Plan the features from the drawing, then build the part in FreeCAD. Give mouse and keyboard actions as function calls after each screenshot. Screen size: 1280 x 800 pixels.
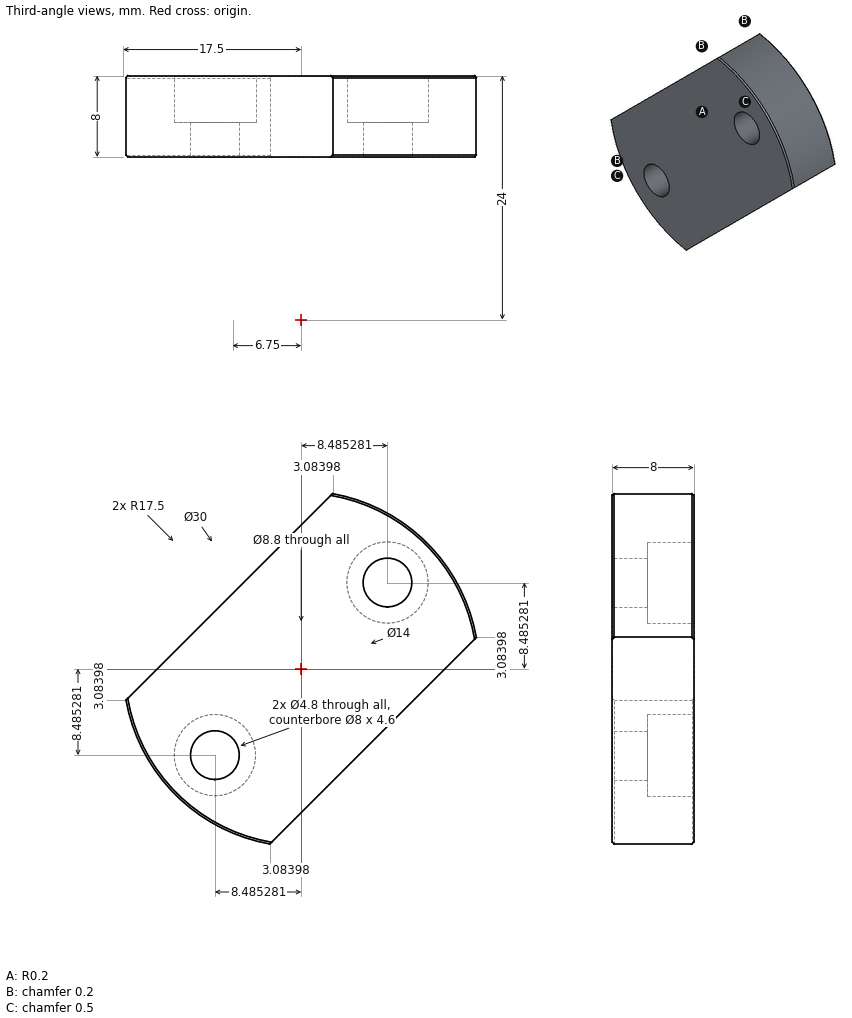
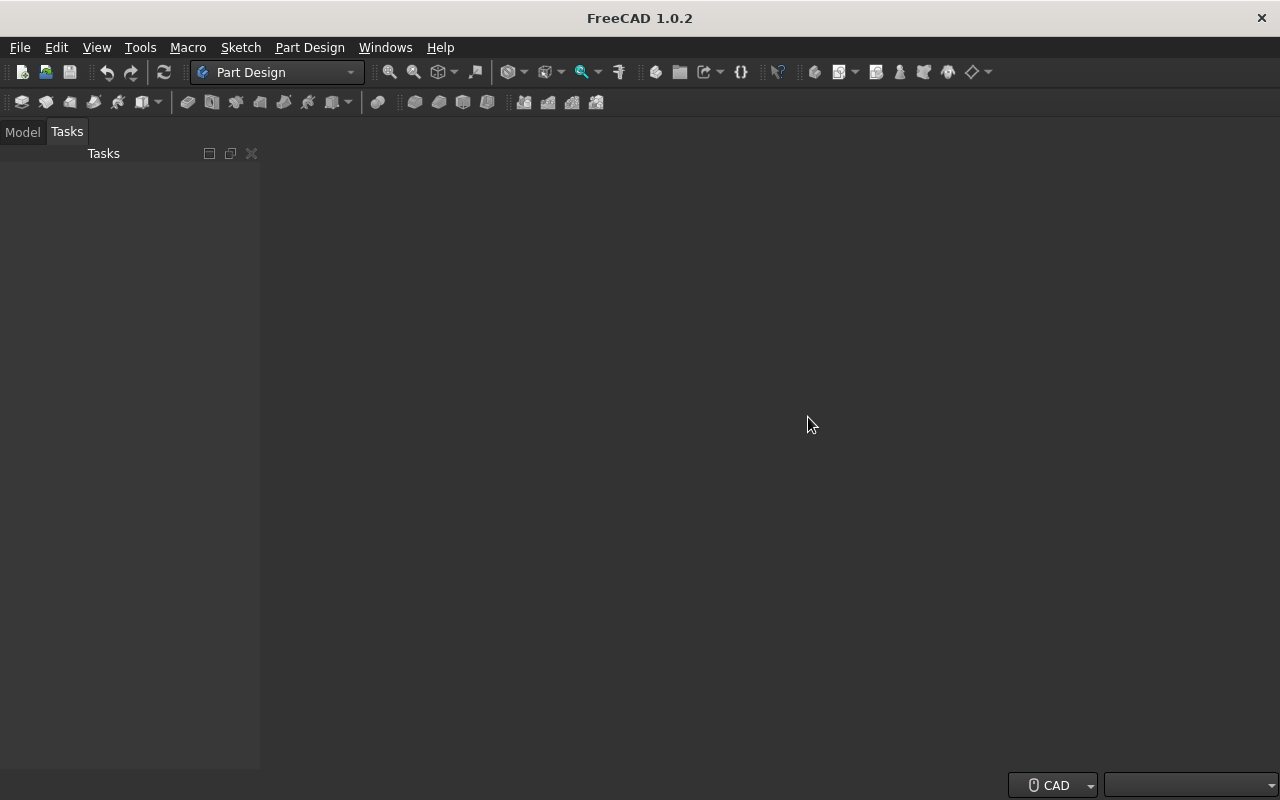
click(22, 72)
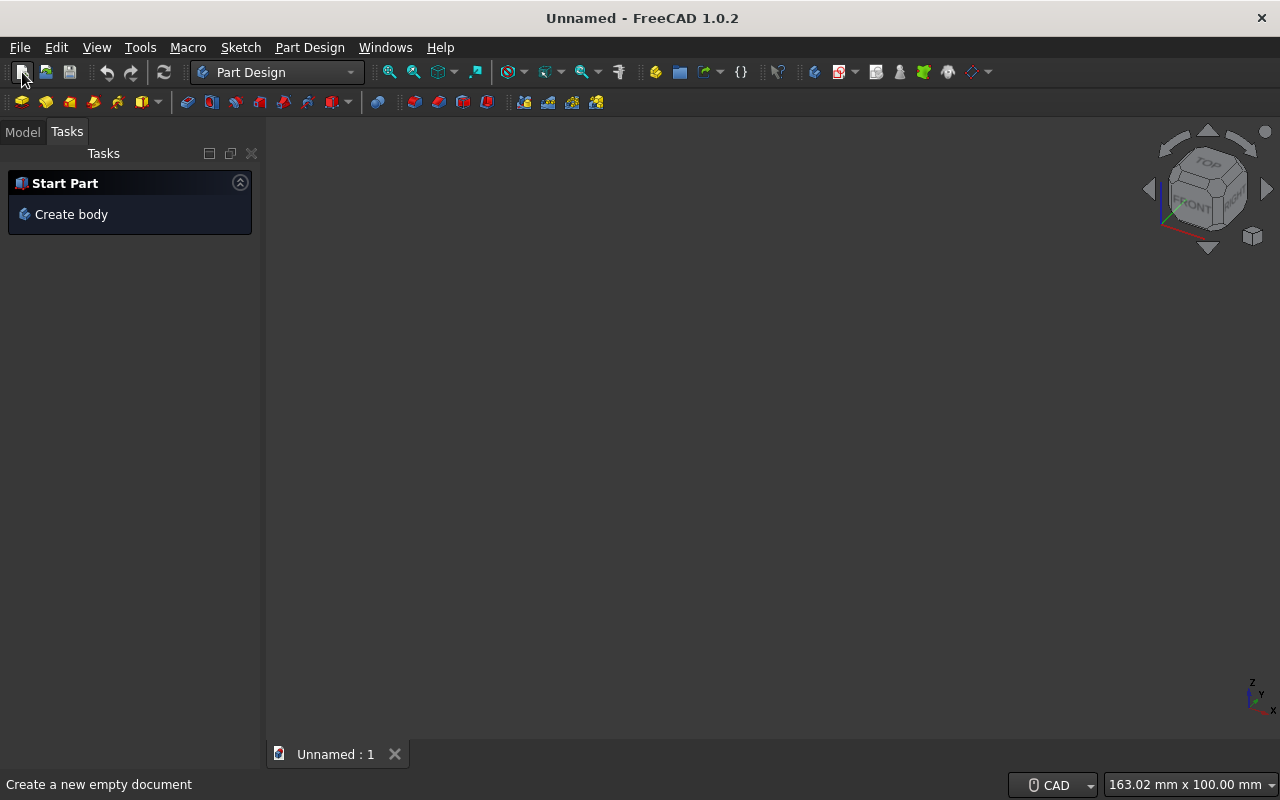
click(840, 72)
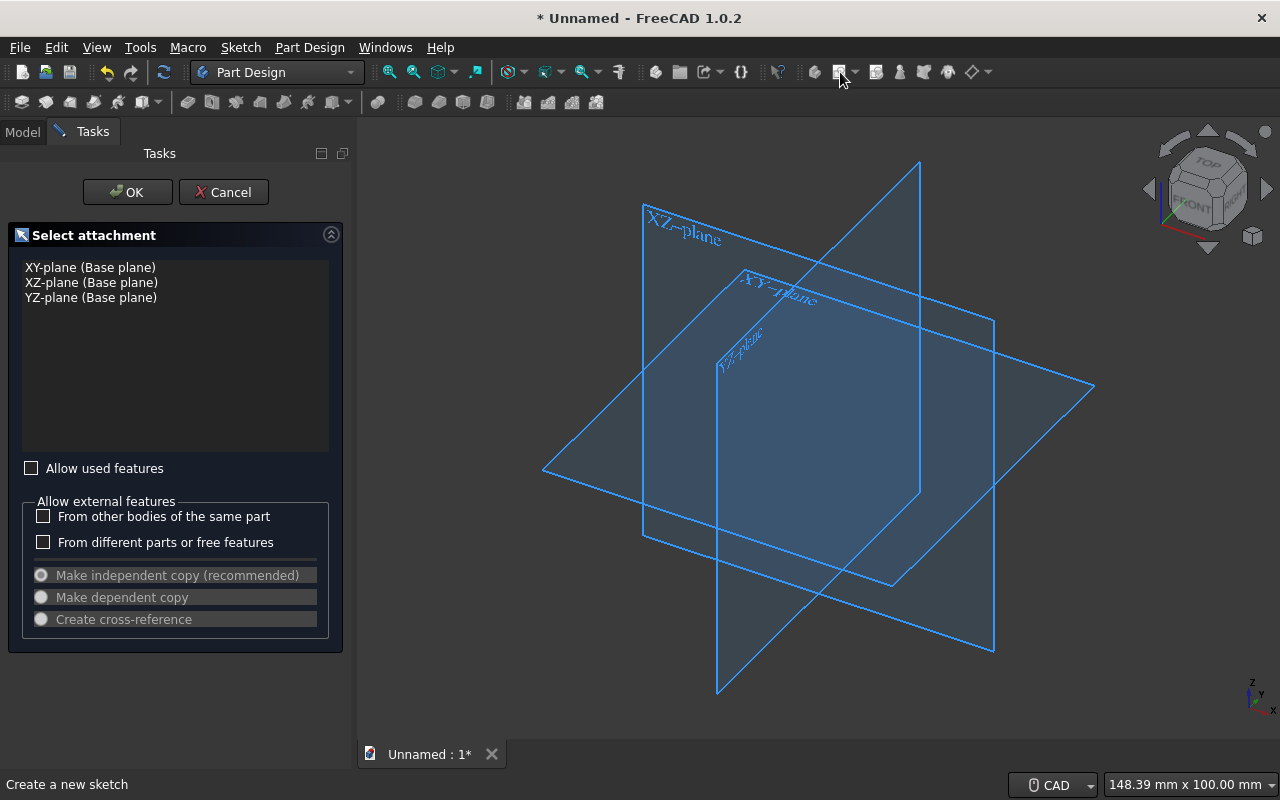
click(82, 268)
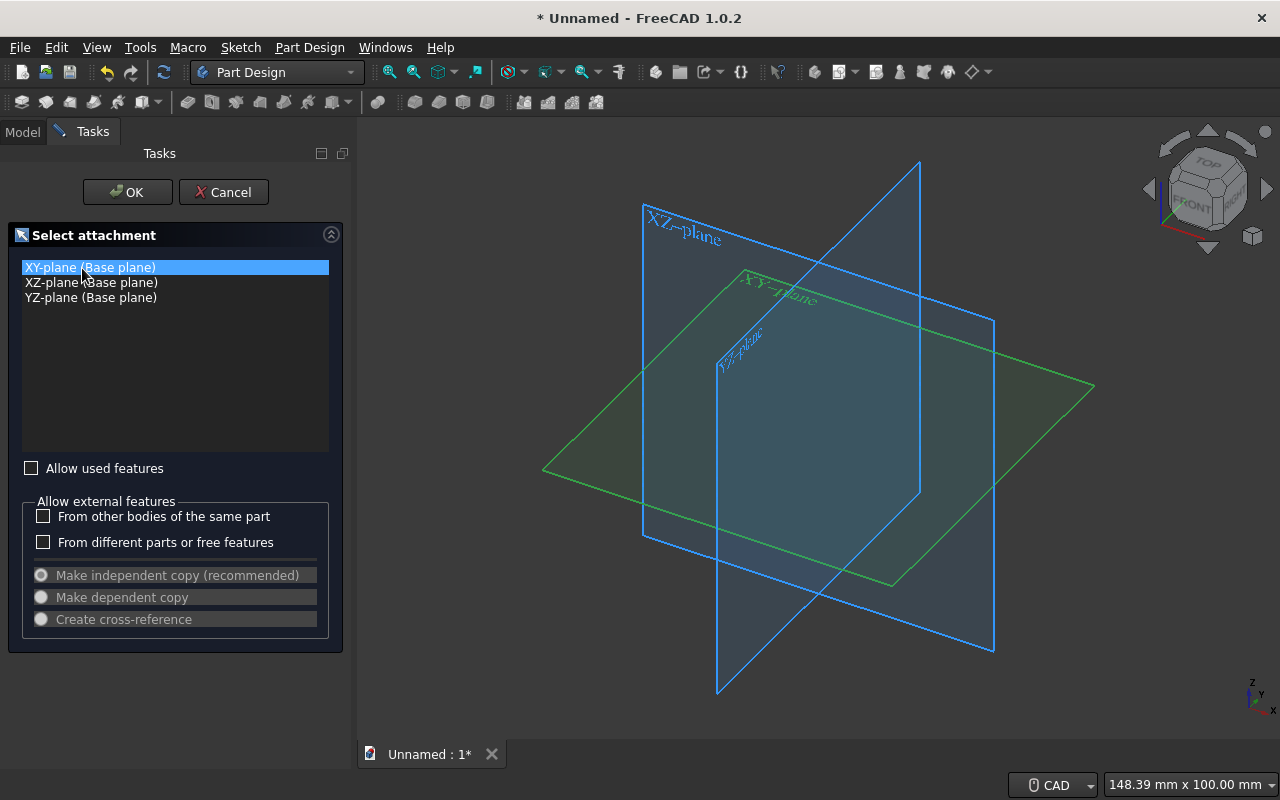
click(128, 192)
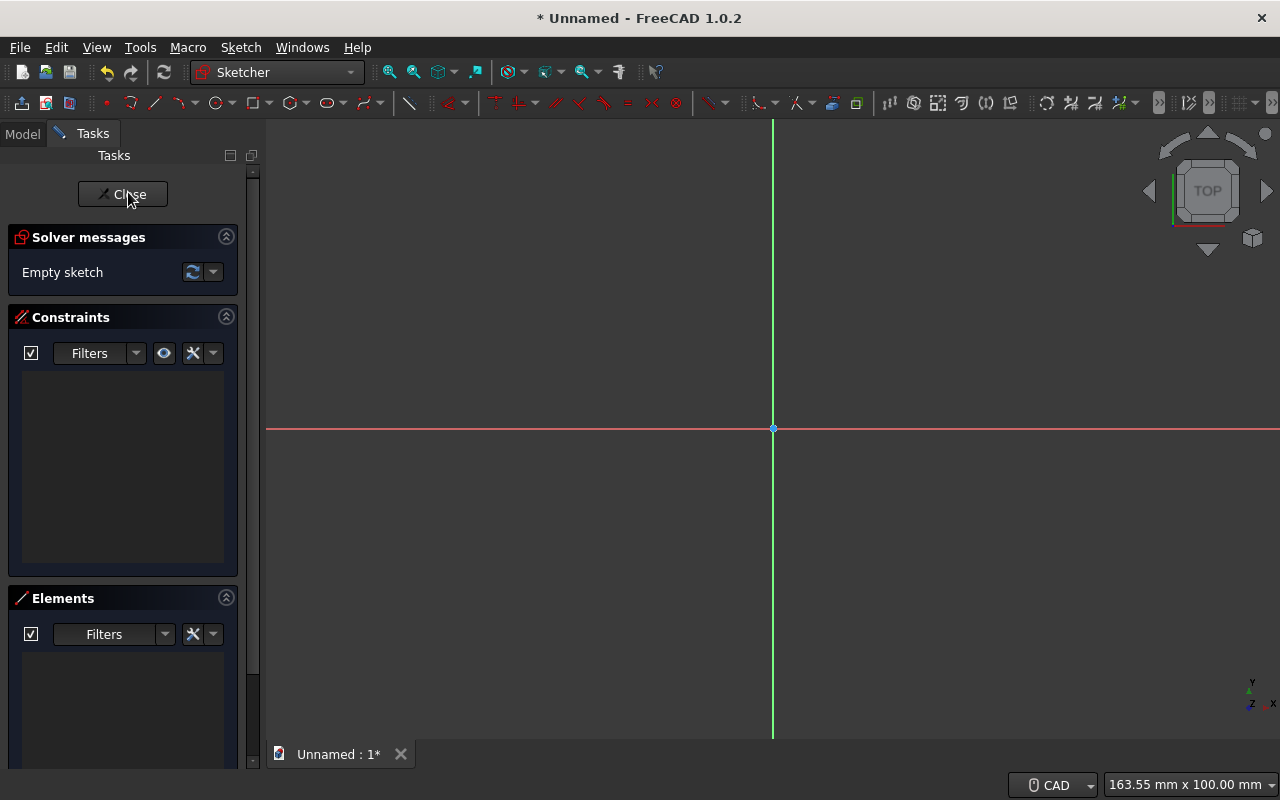
scroll(727, 311, up, 5)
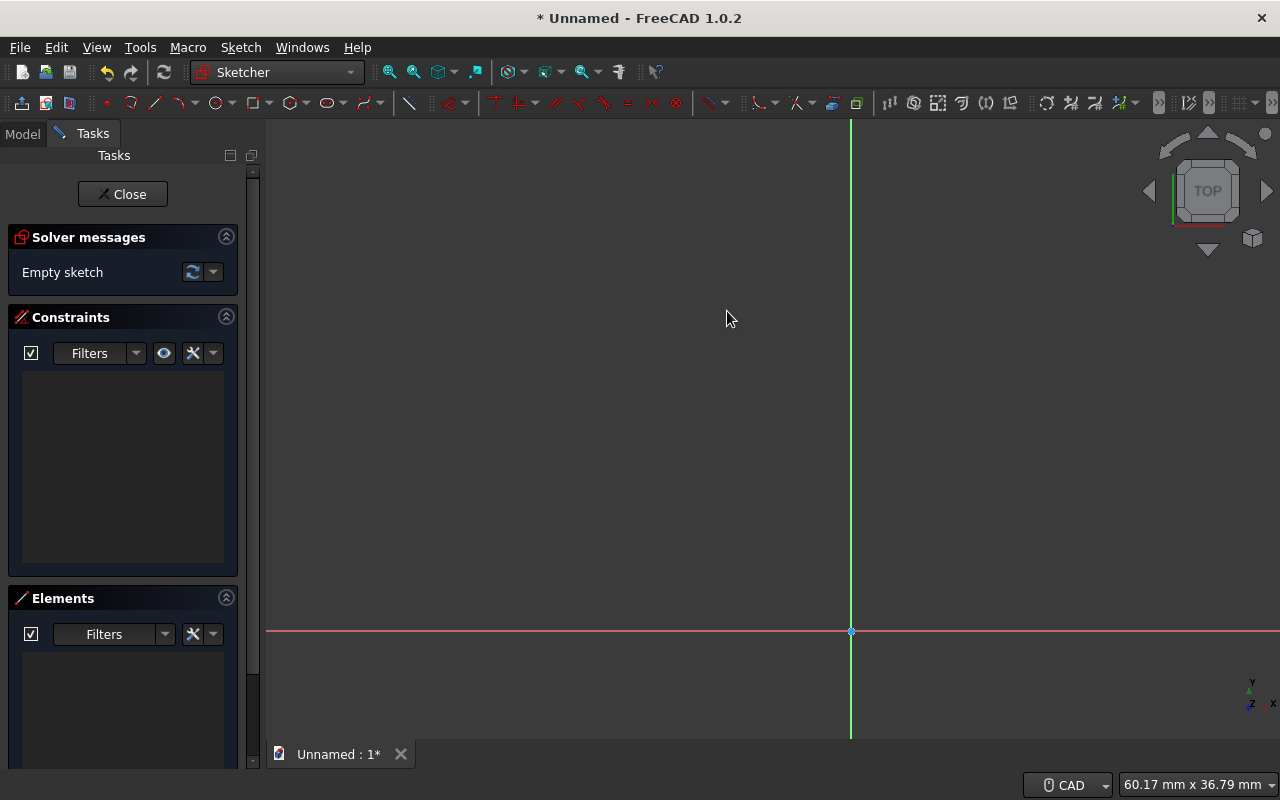
click(132, 104)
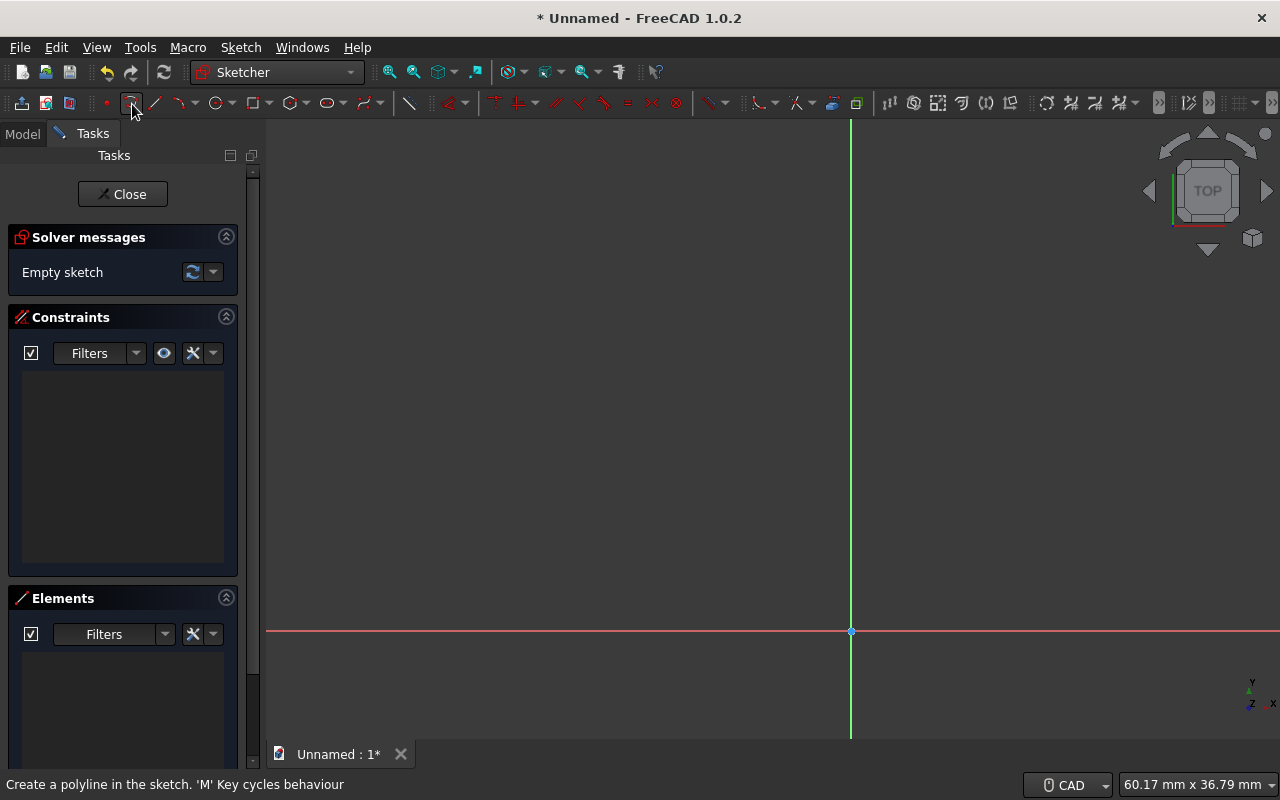
click(851, 631)
click(842, 227)
click(556, 227)
click(556, 362)
click(737, 362)
click(737, 622)
click(851, 631)
key(Escape)
key(Escape)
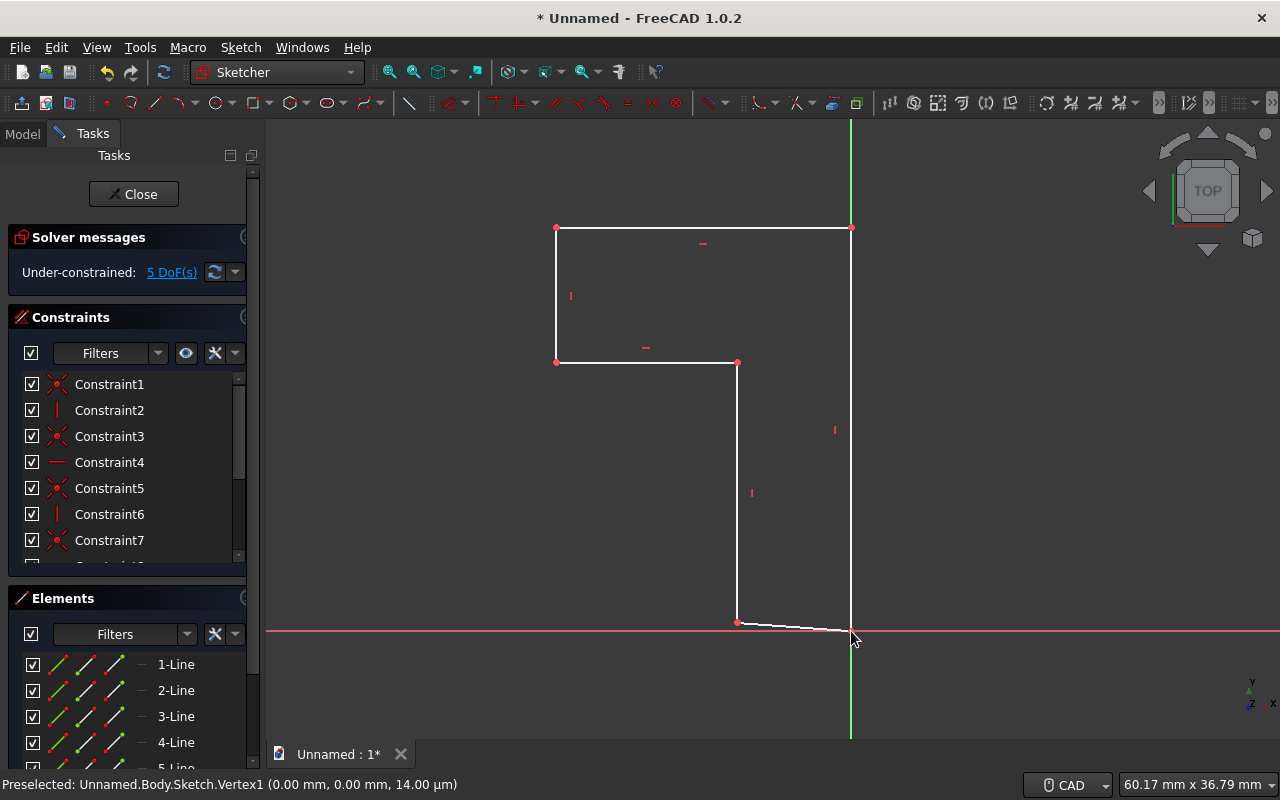
click(817, 629)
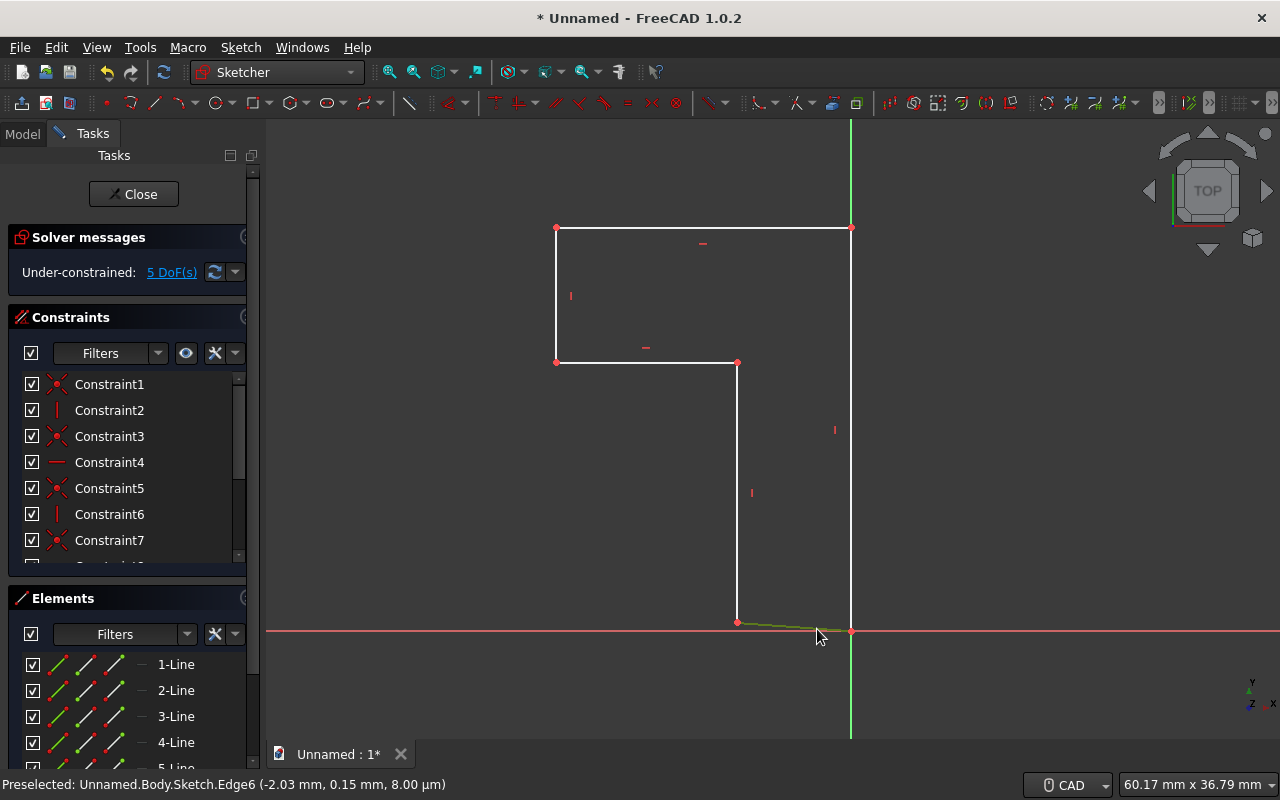
key(h)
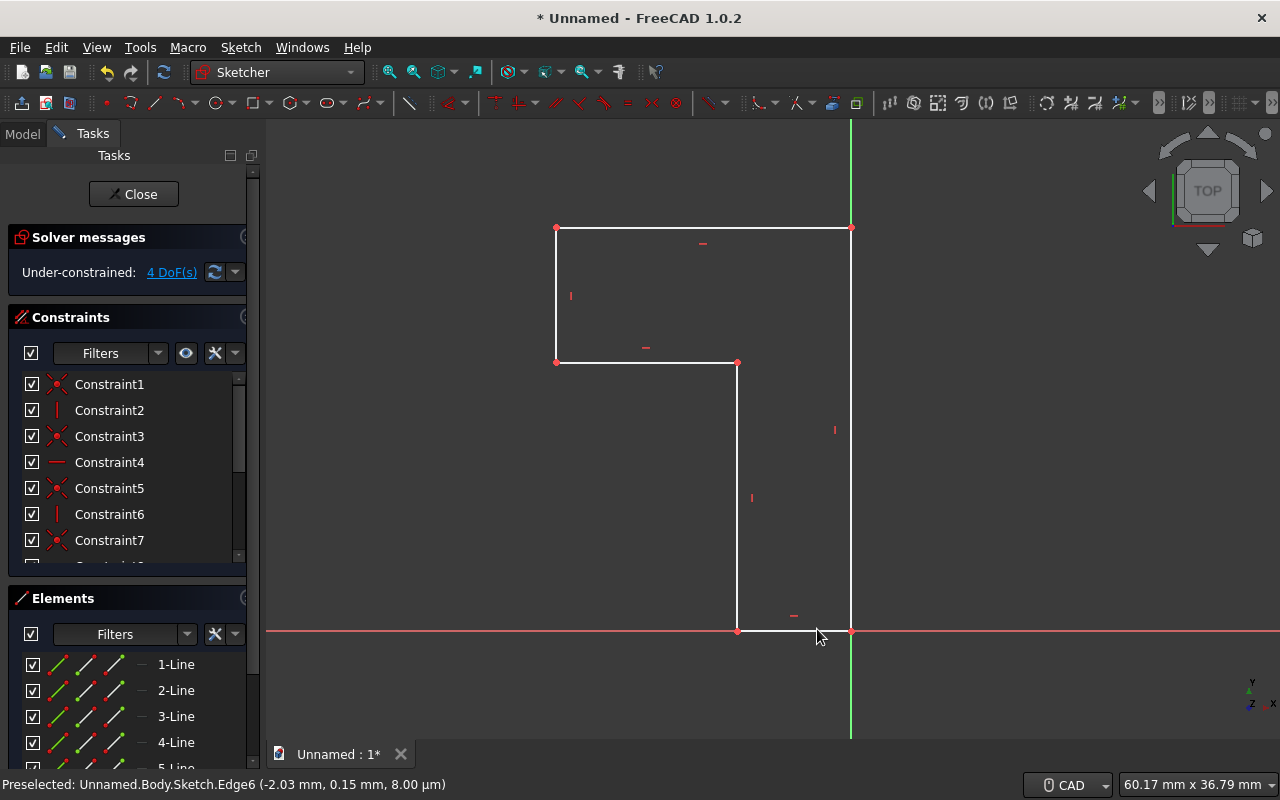
click(556, 269)